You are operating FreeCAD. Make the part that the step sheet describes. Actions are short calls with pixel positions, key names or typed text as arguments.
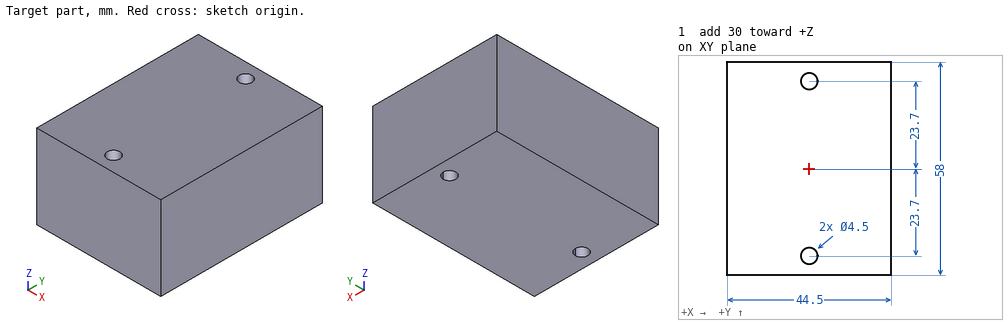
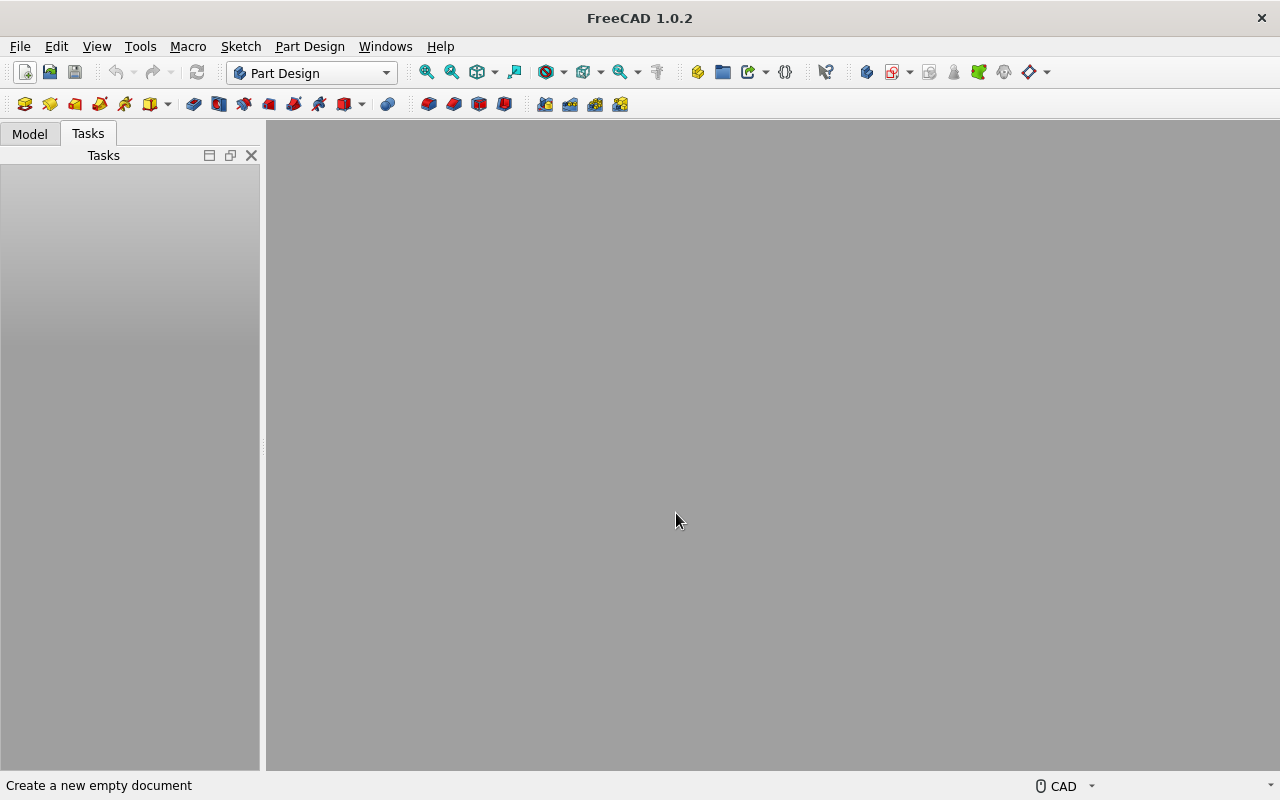
click(25, 72)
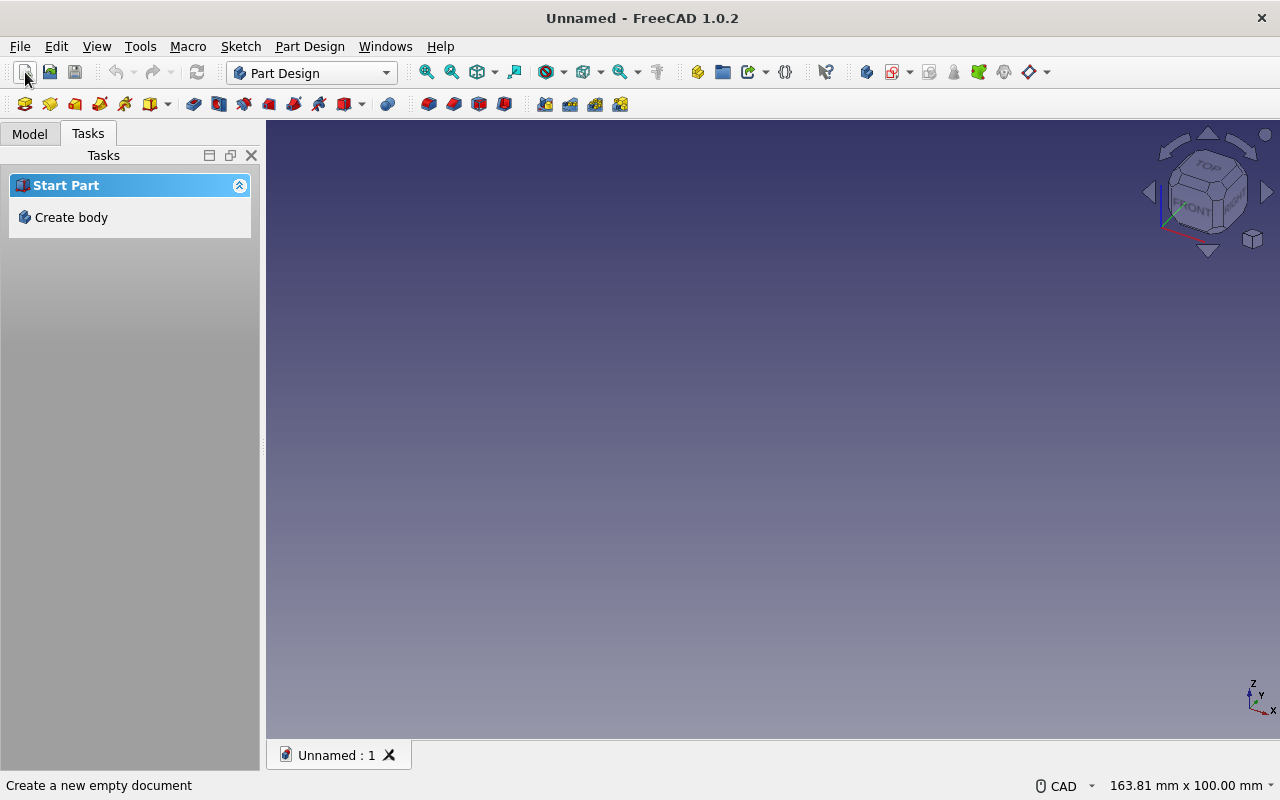
click(892, 72)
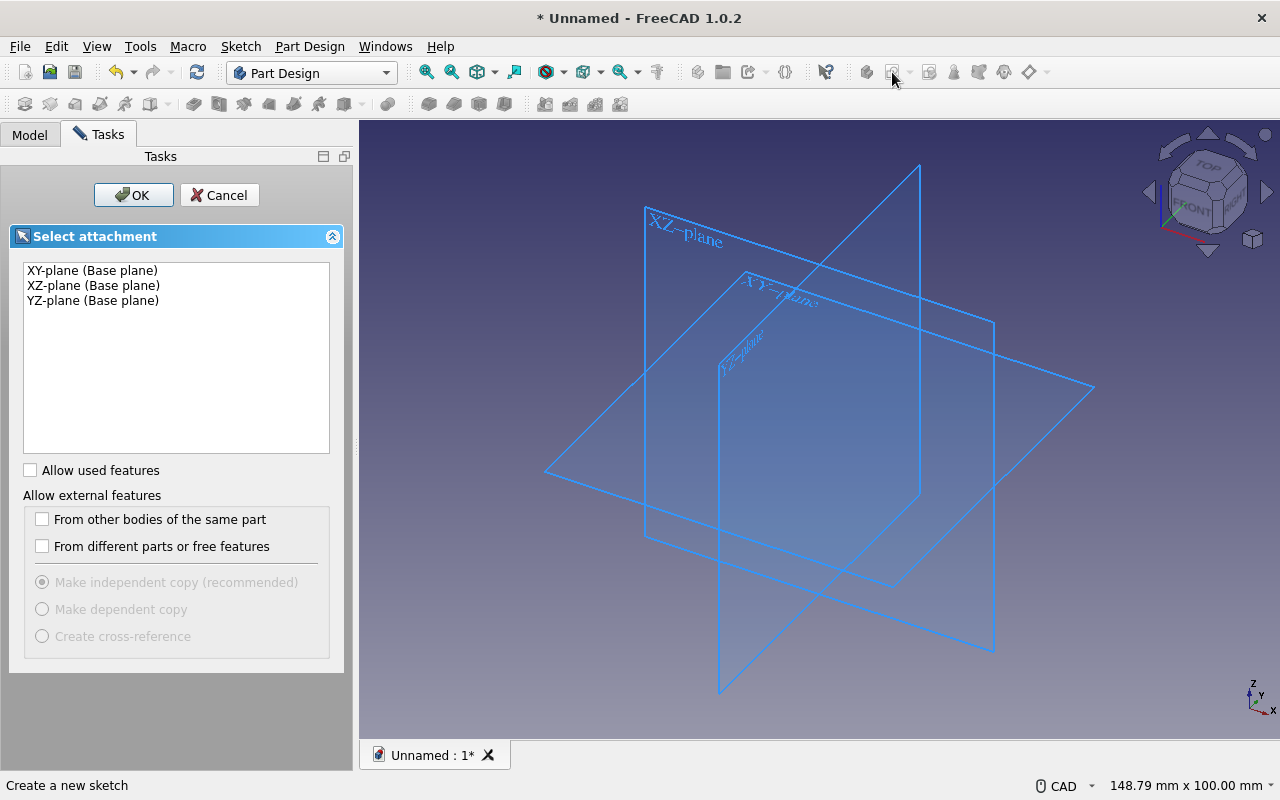
click(84, 270)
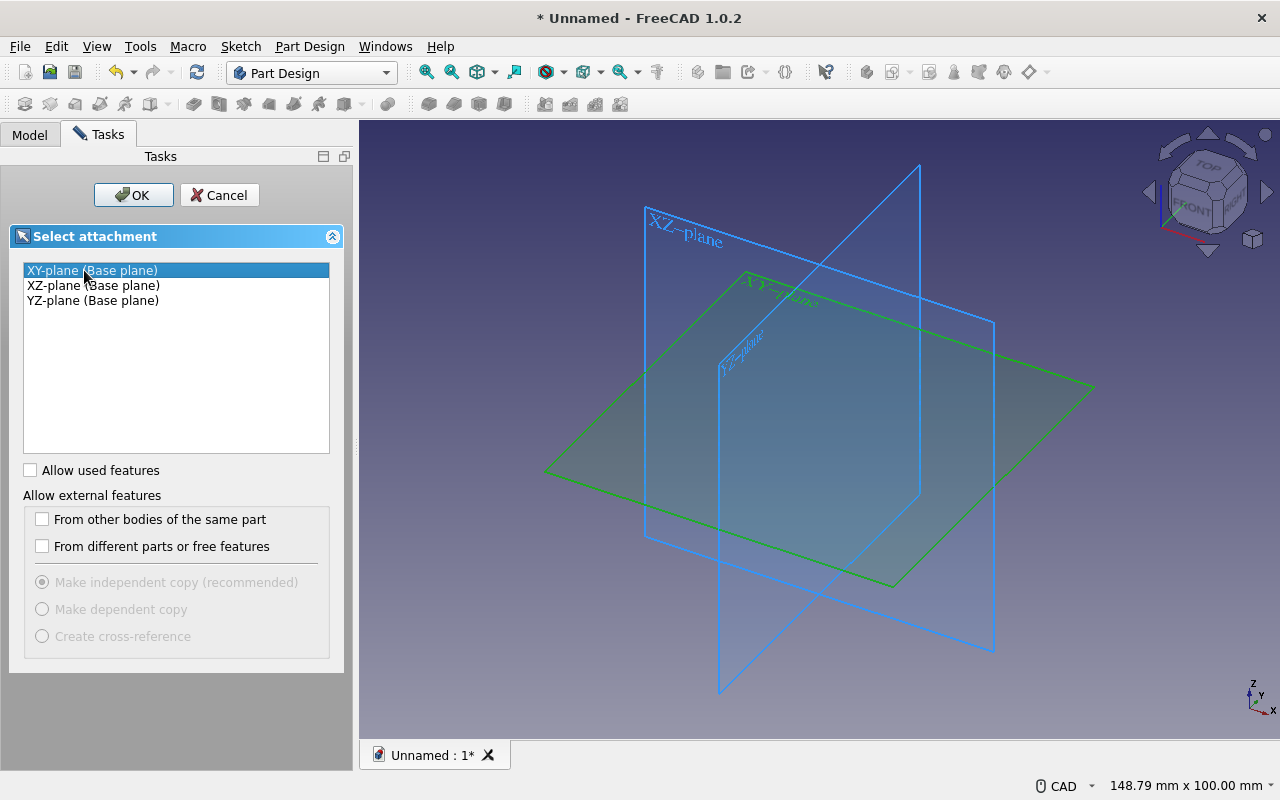
click(134, 195)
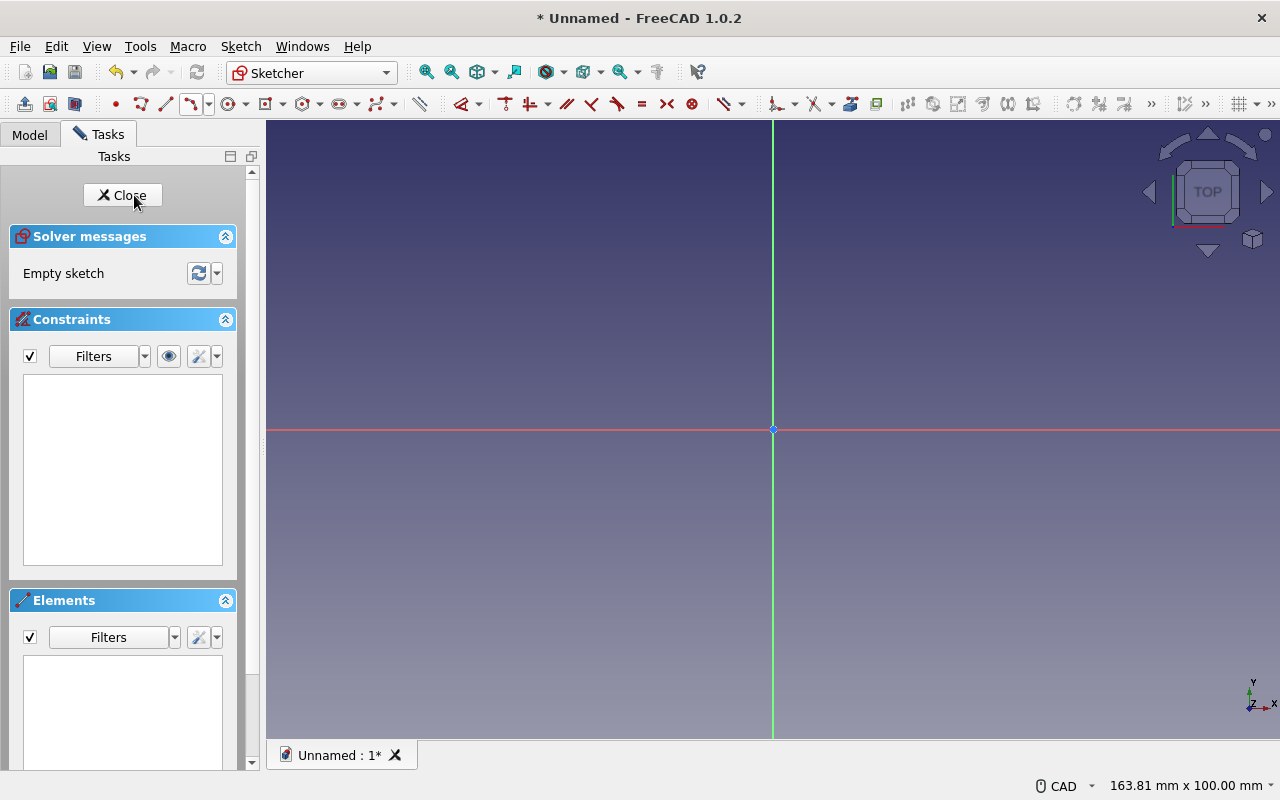
key(g)
key(v)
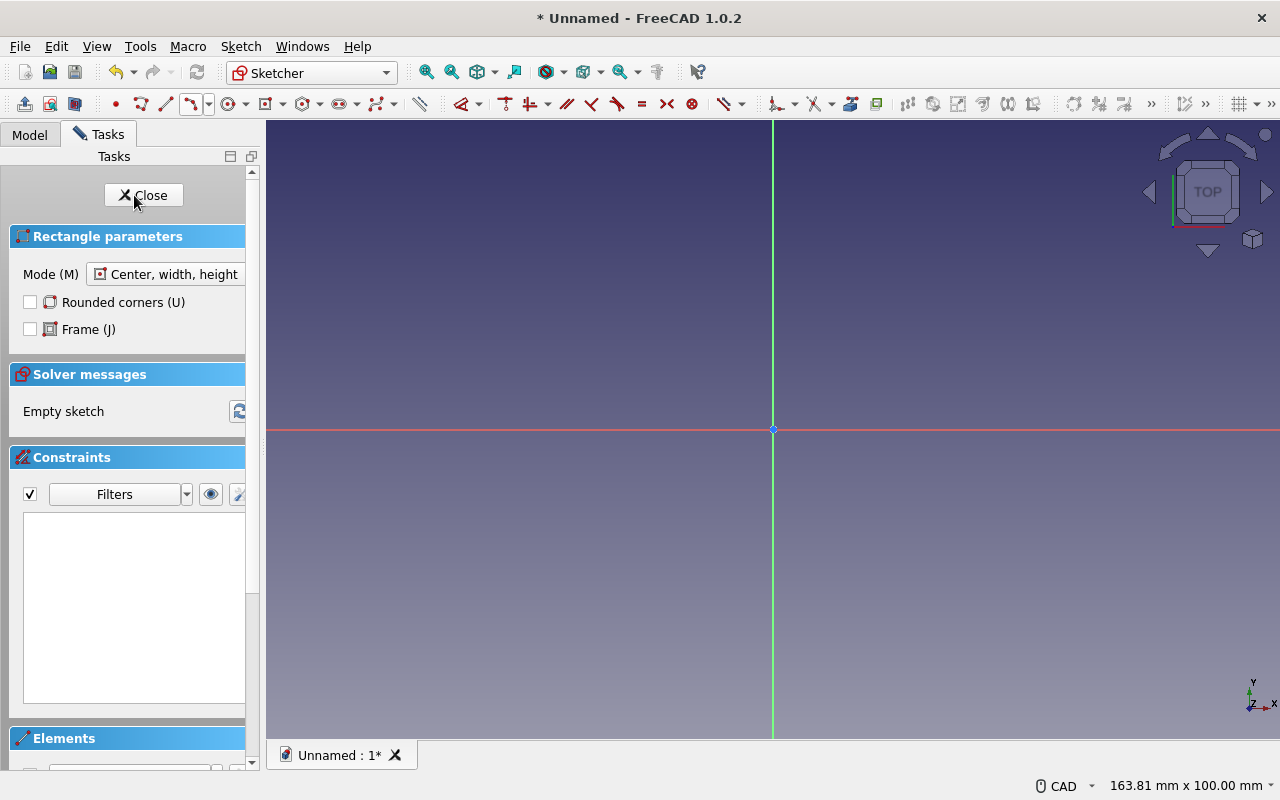
click(773, 430)
click(911, 250)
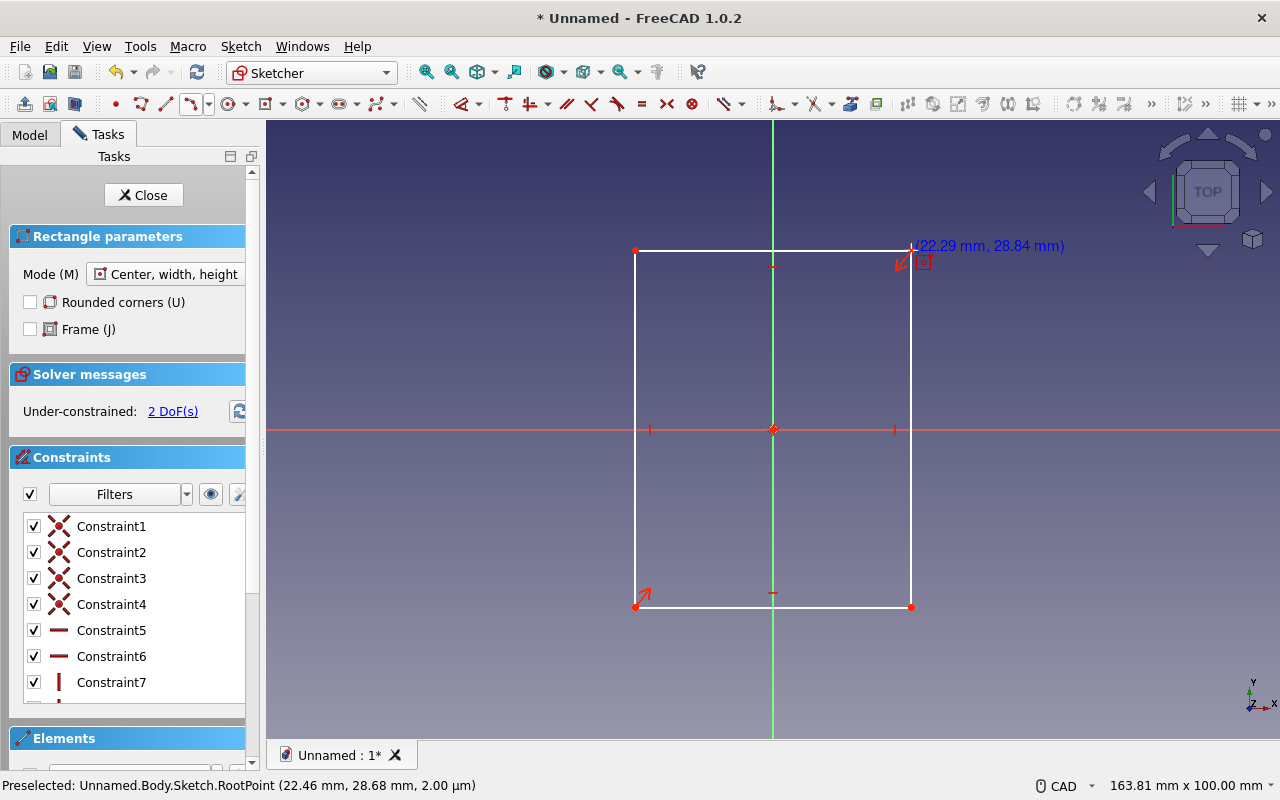
click(228, 104)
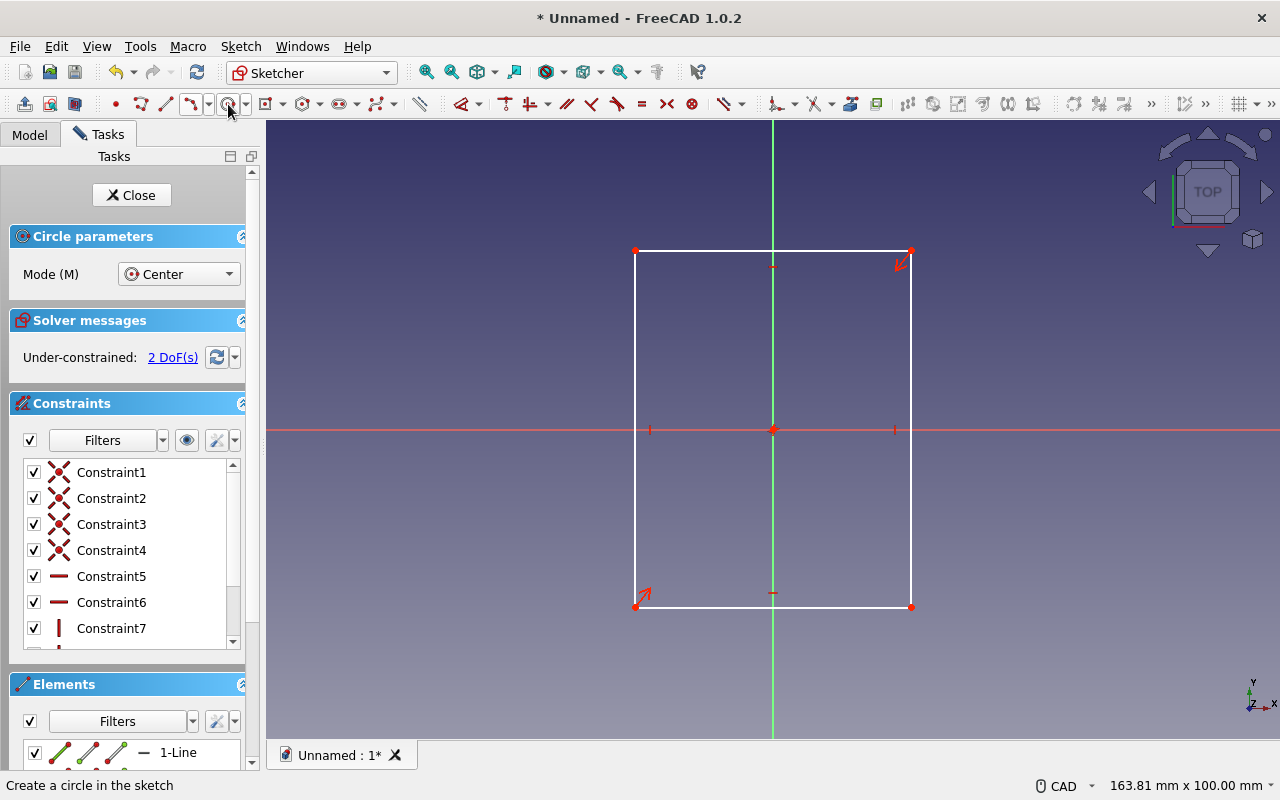
scroll(773, 576, up, 3)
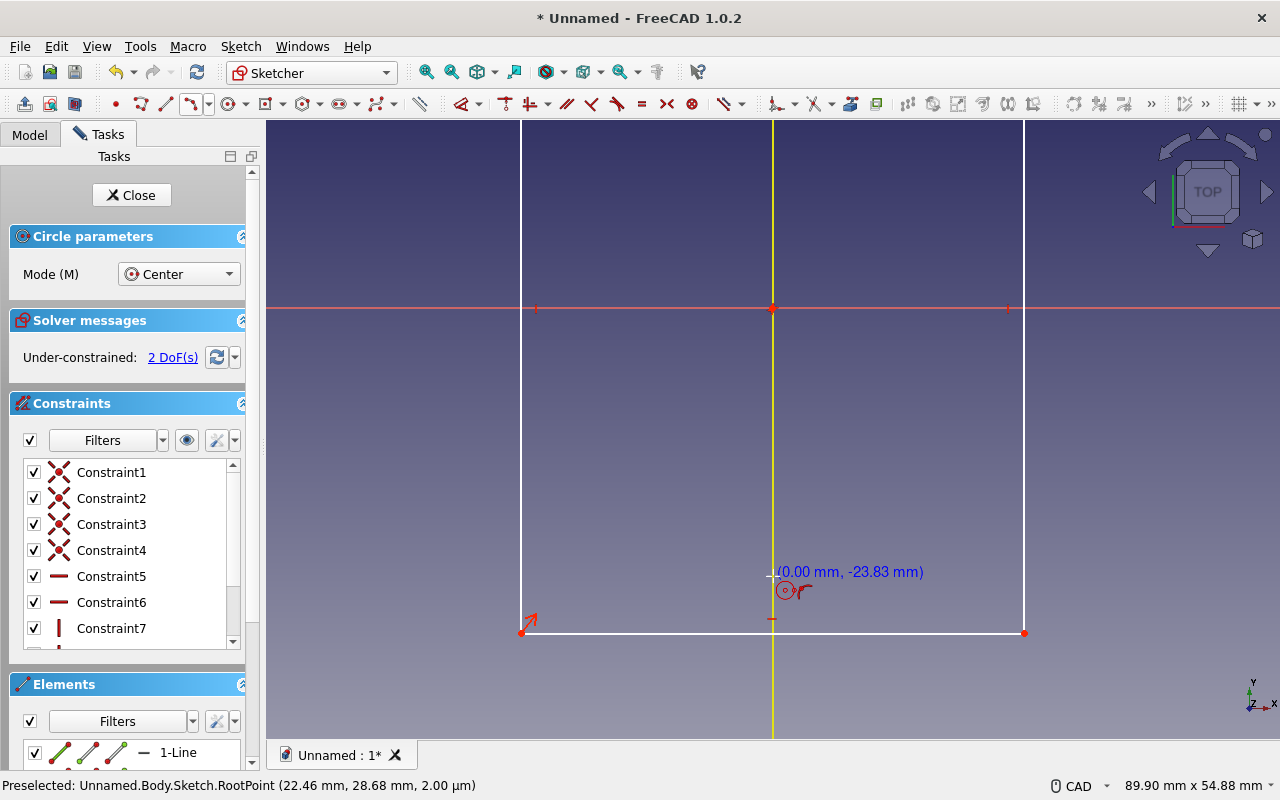
click(773, 576)
click(791, 558)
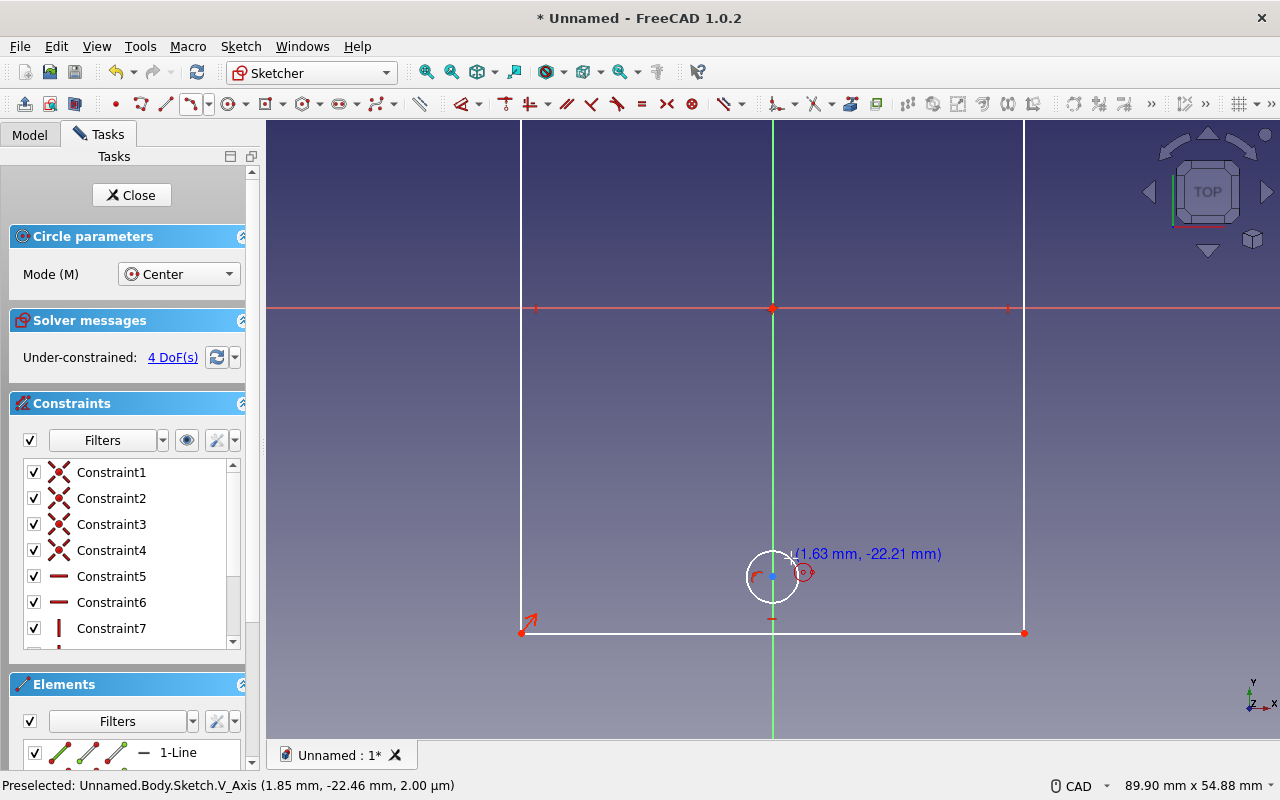
scroll(566, 676, down, 2)